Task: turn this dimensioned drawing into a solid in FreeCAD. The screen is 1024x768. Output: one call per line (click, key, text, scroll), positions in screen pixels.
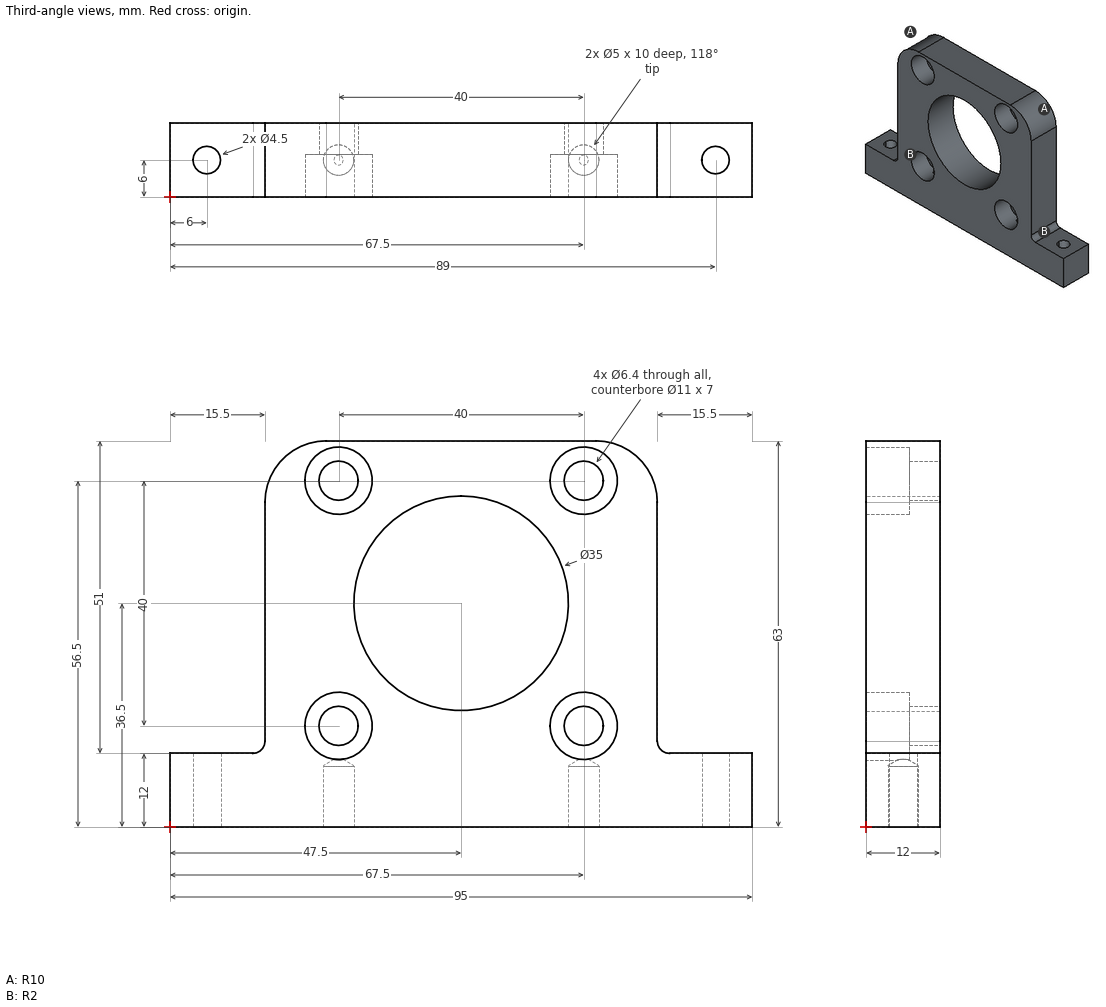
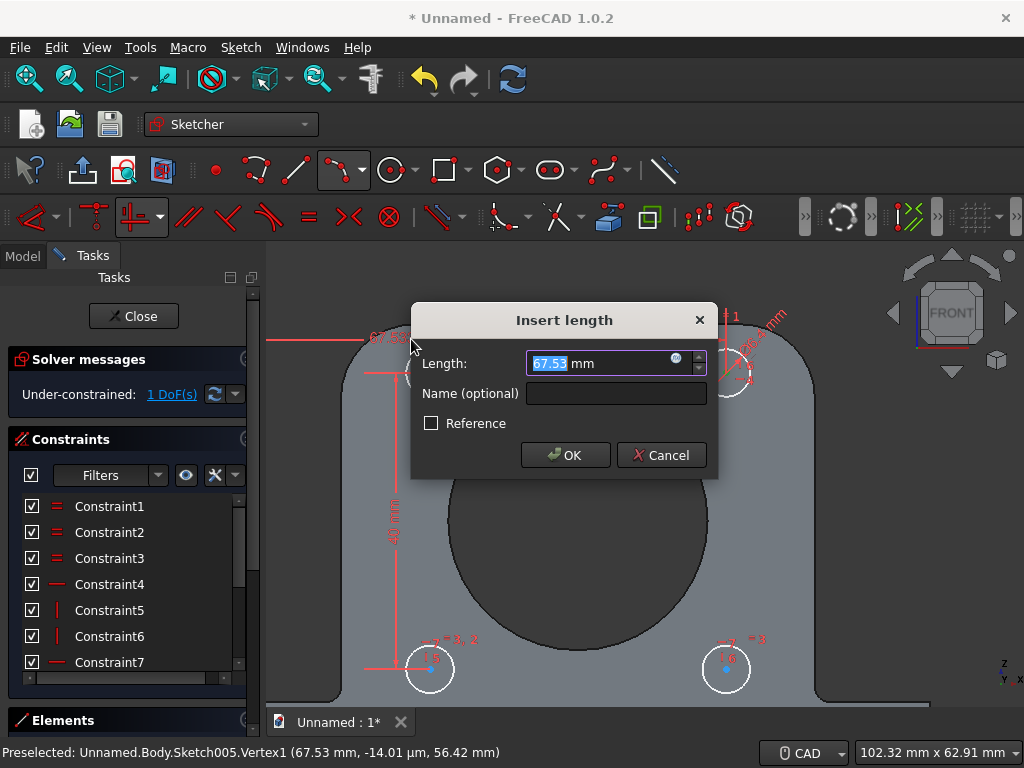
text(67.5)
key(Return)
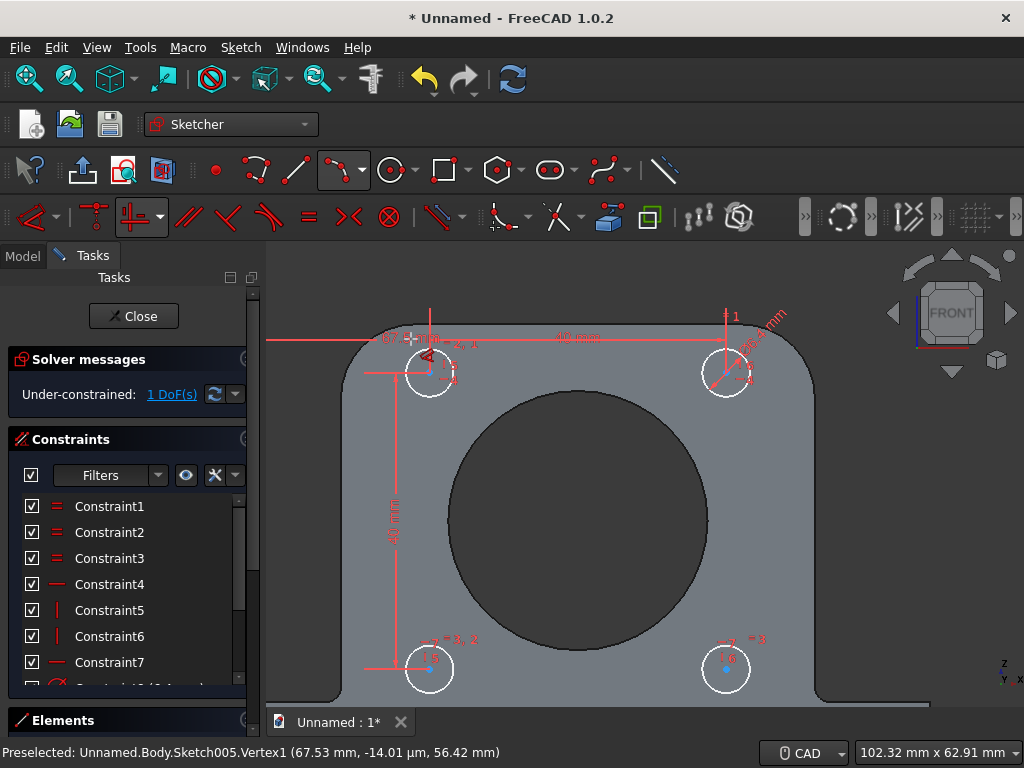
click(726, 373)
click(760, 526)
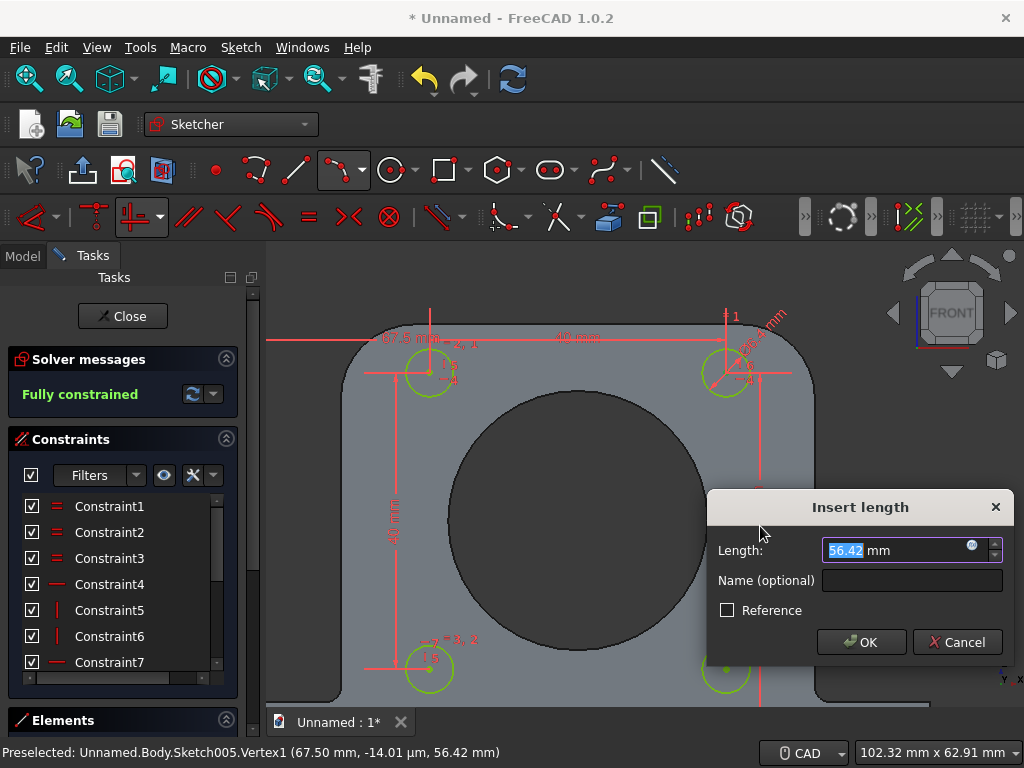
text(56.5)
key(Return)
key(Escape)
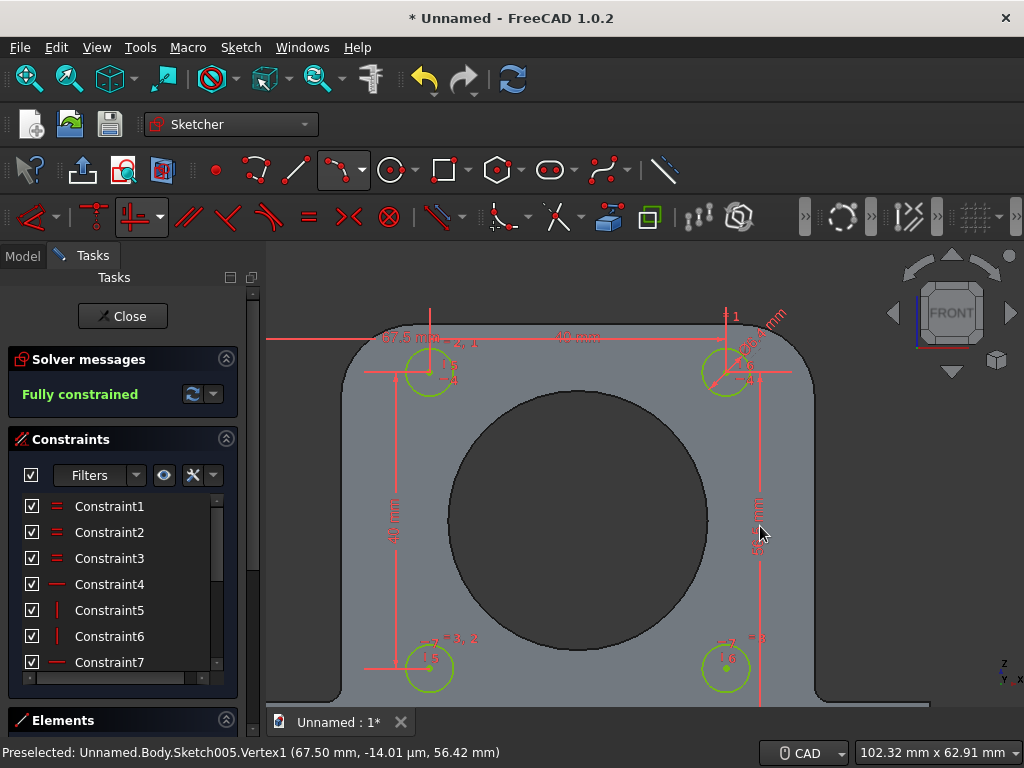
click(123, 316)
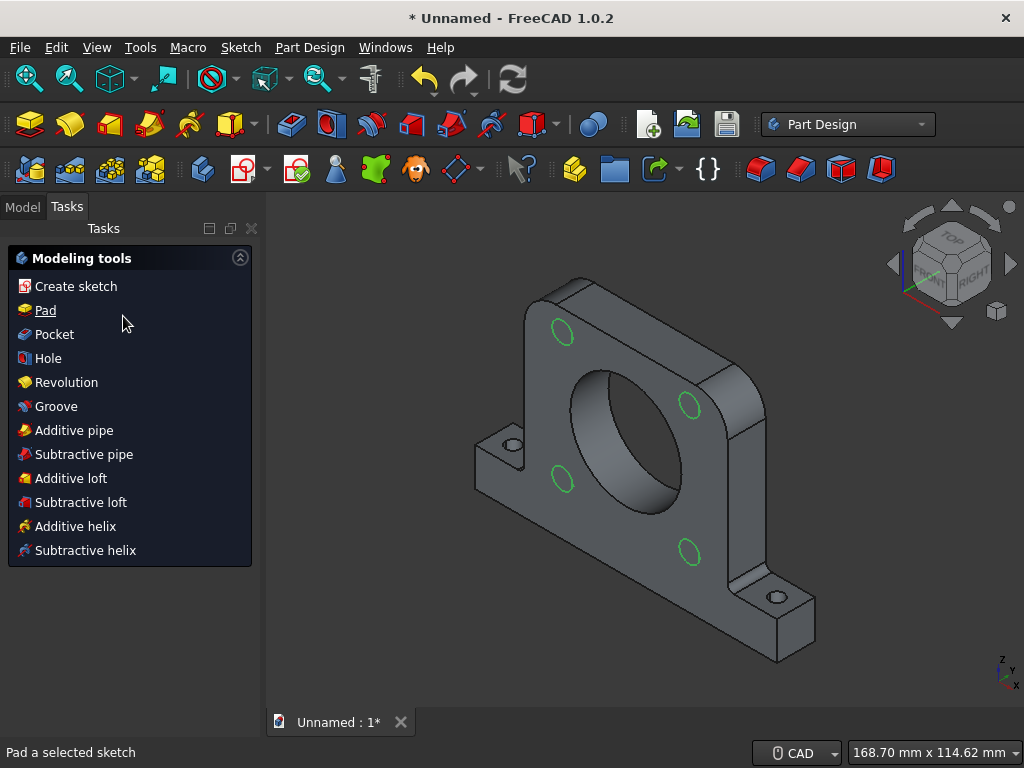
click(332, 124)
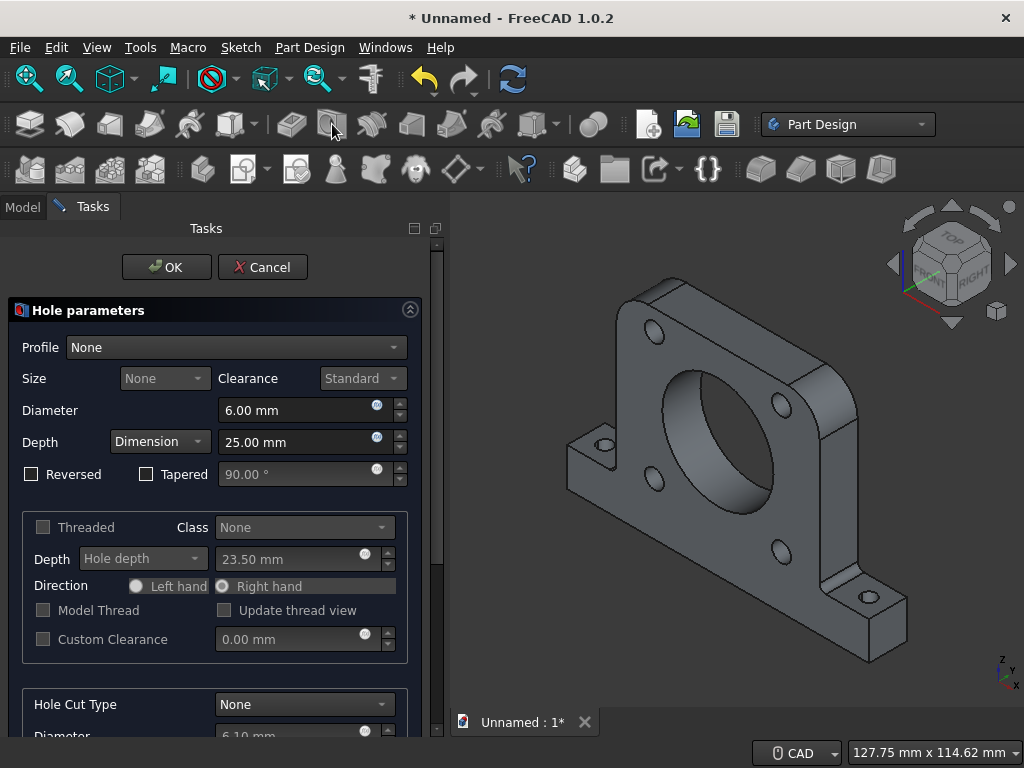
triple_click(305, 410)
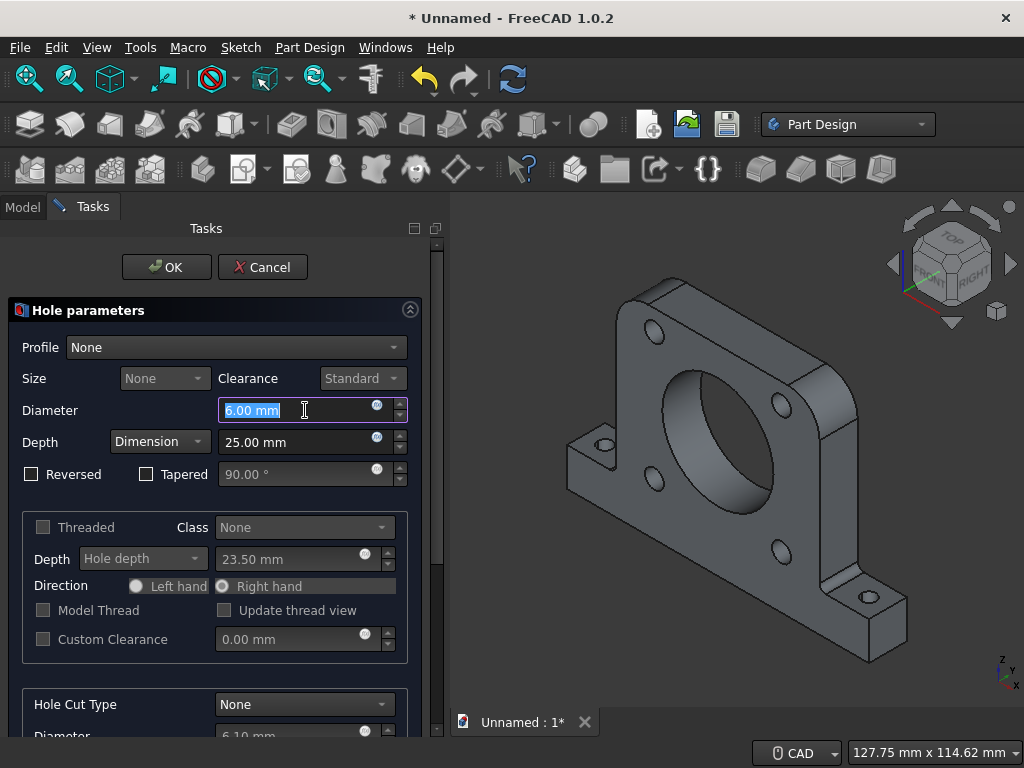
text(6.4)
key(Tab)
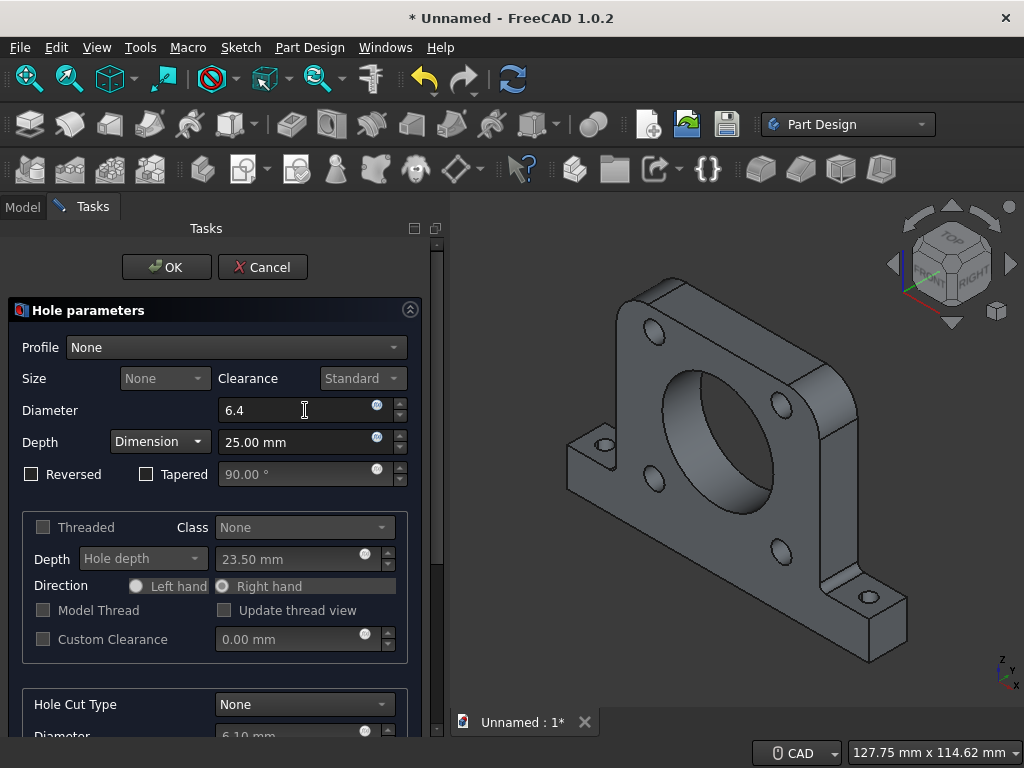
click(161, 442)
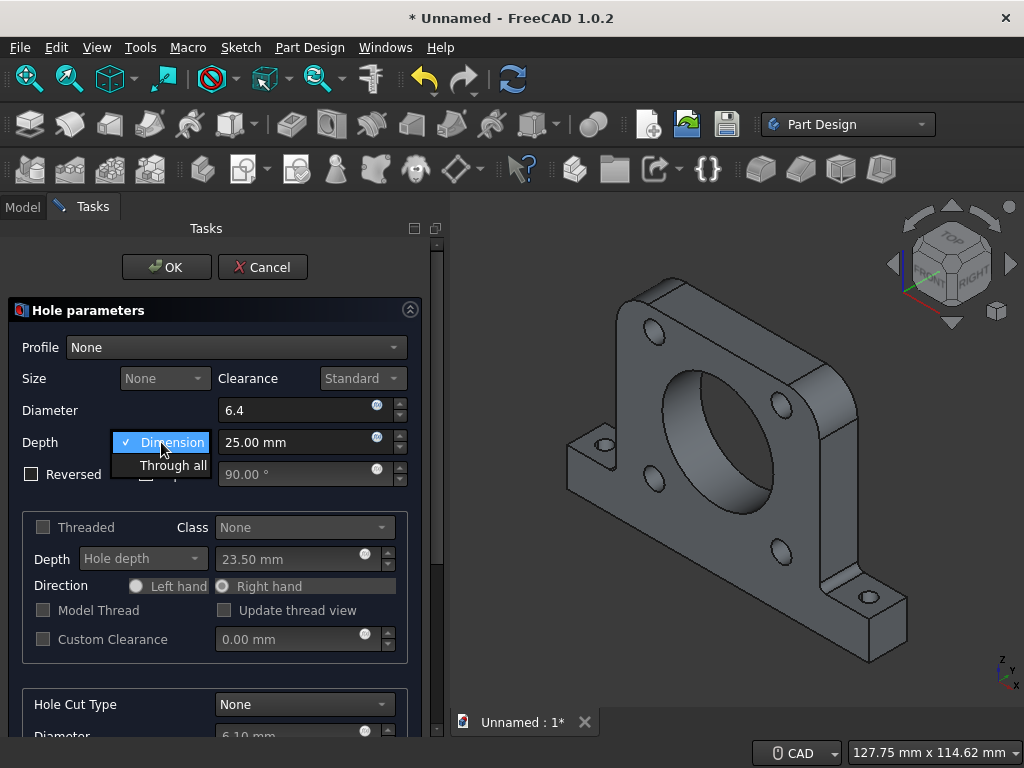
click(160, 466)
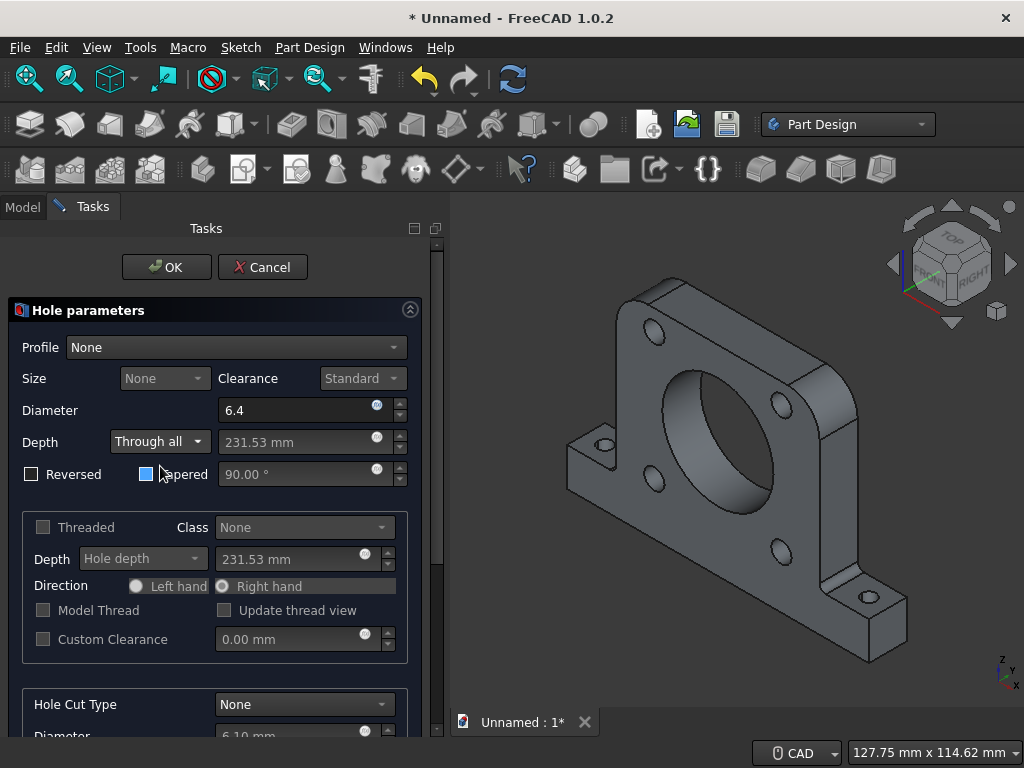
click(306, 704)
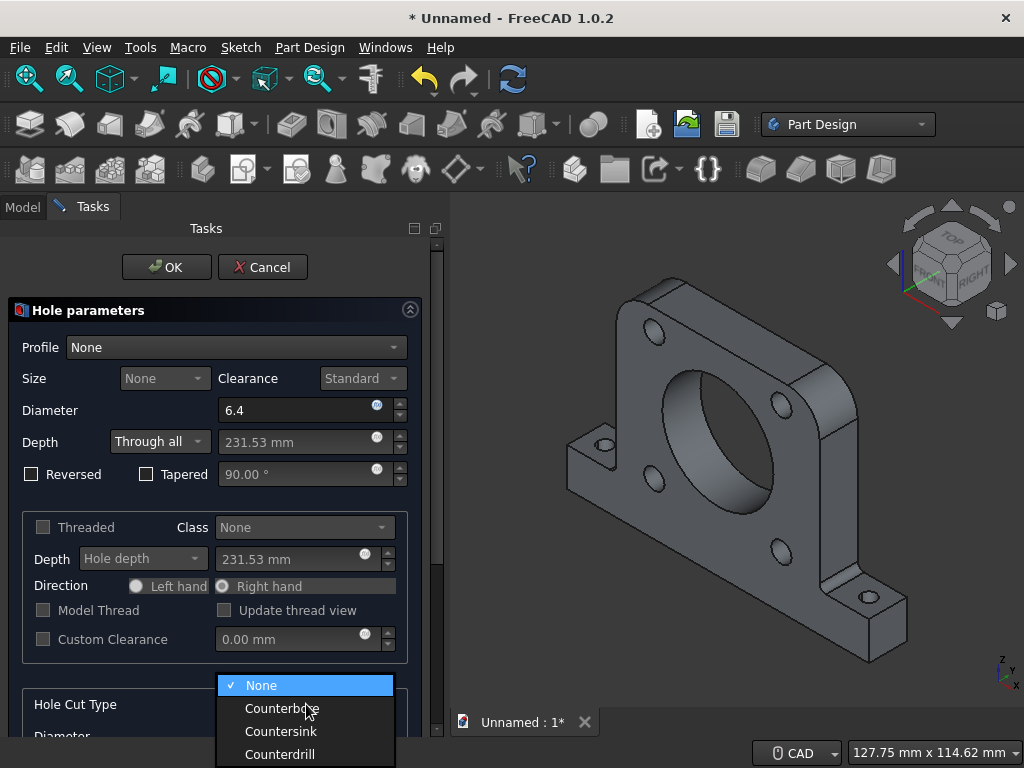
click(304, 708)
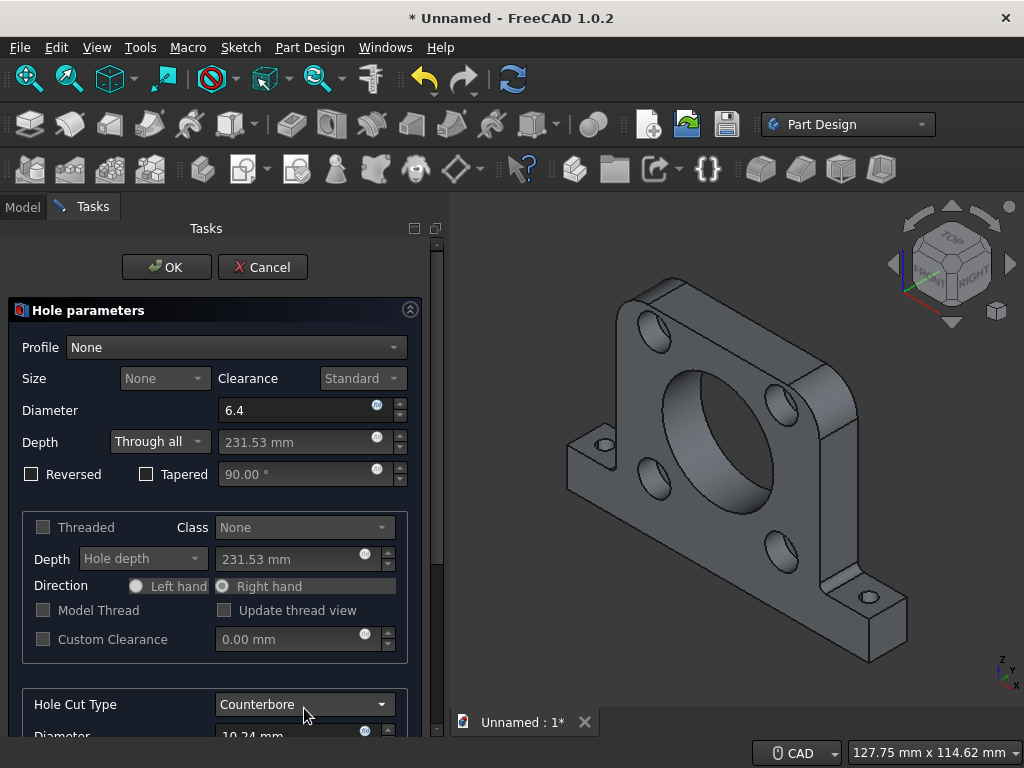
scroll(437, 487, down, 2)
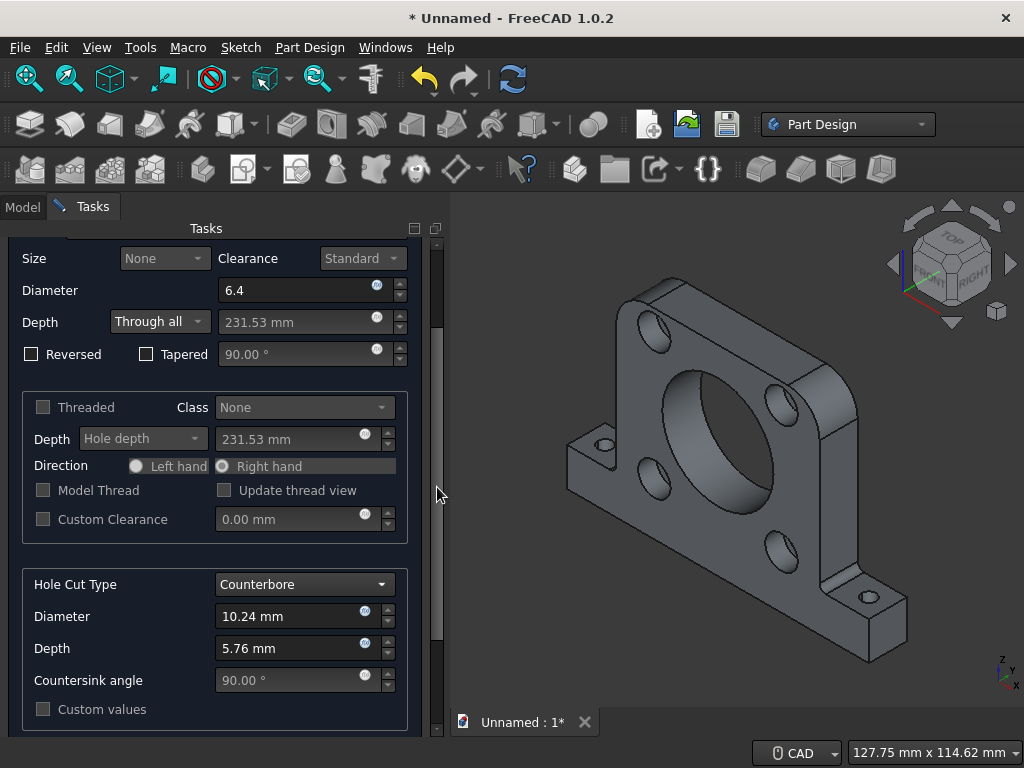
triple_click(298, 616)